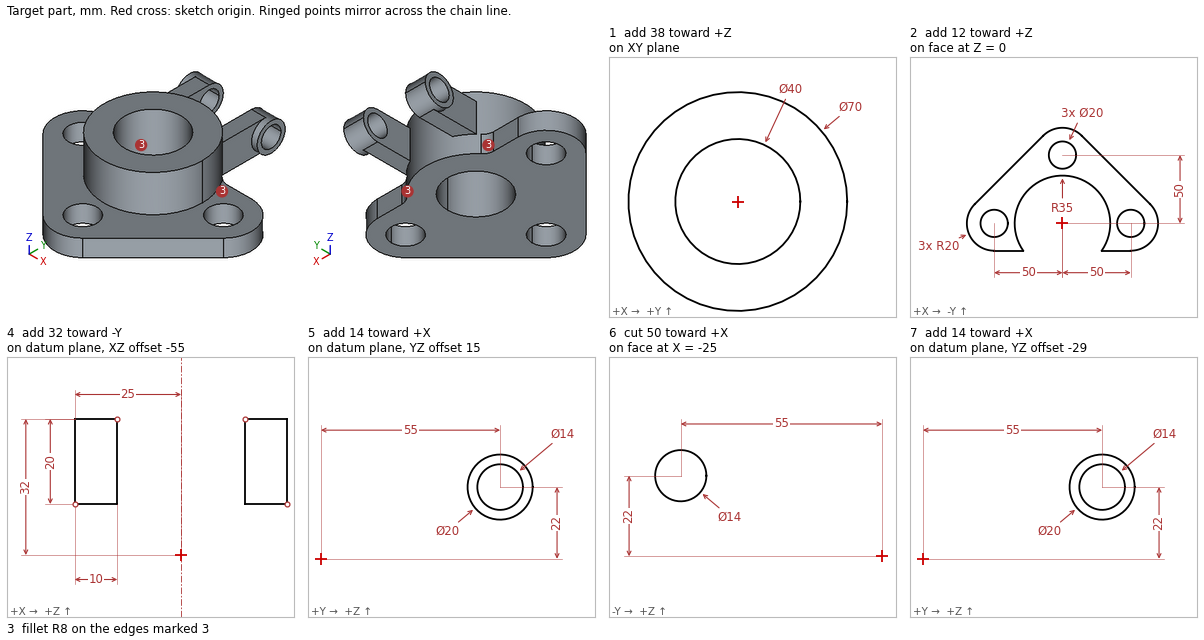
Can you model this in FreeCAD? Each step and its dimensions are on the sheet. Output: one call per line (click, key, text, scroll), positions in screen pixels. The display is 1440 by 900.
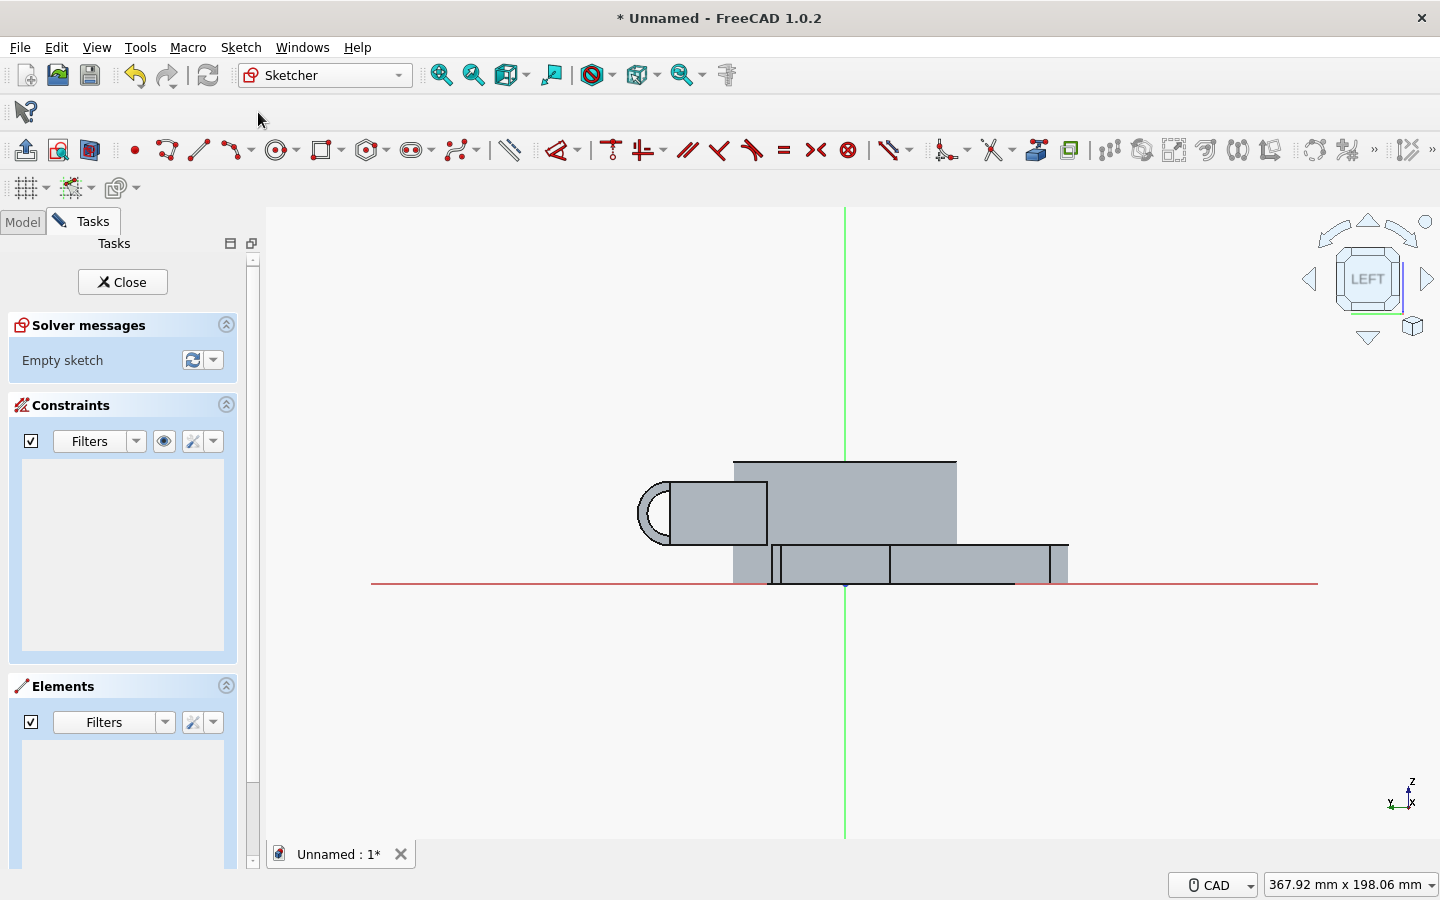
scroll(655, 512, up, 11)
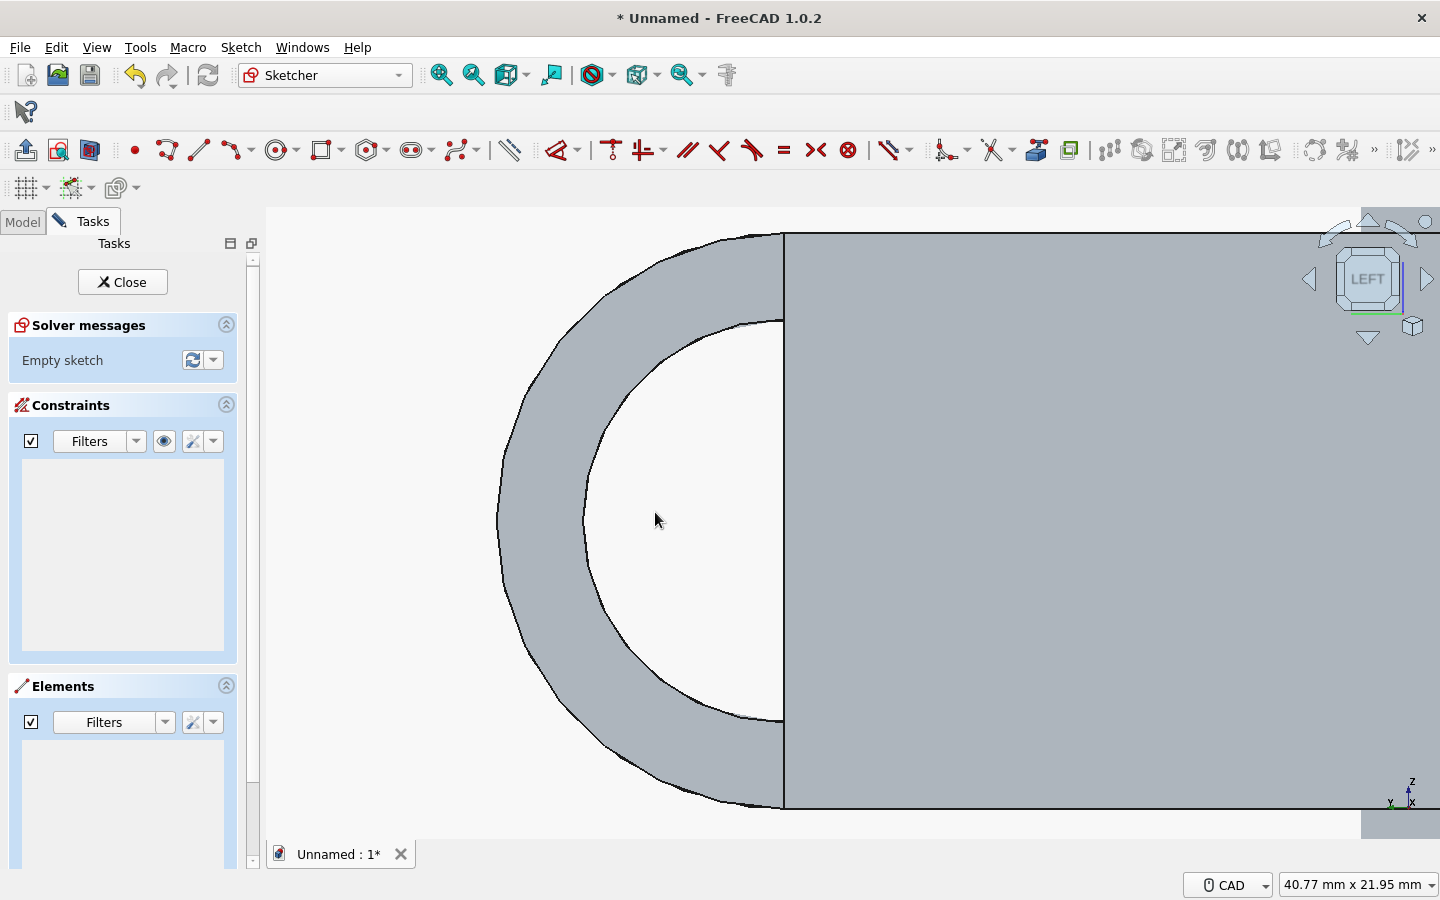
key(g)
key(c)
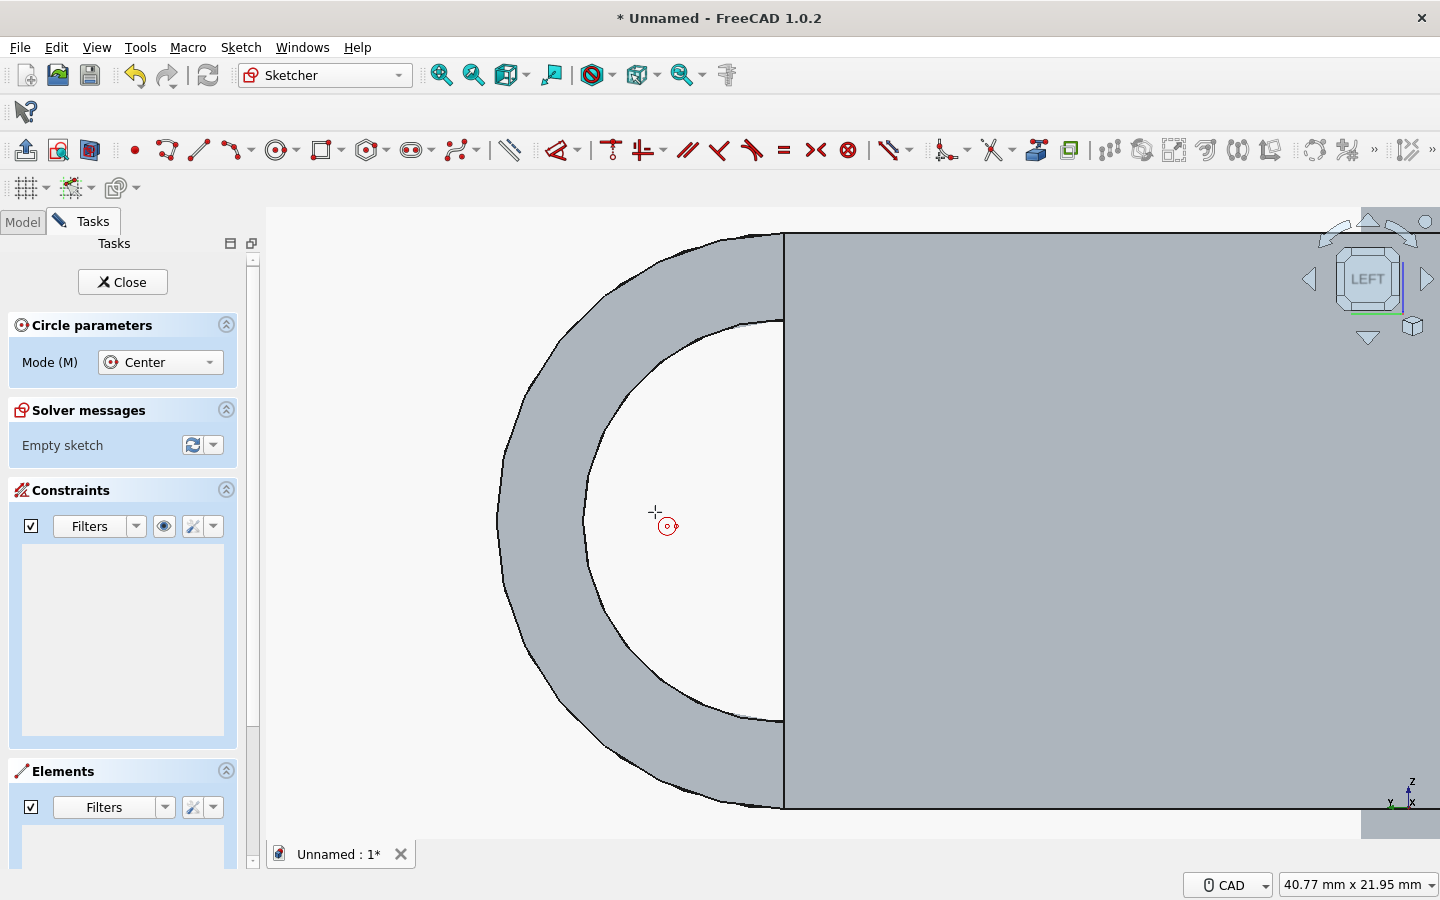
click(784, 521)
click(927, 378)
key(Escape)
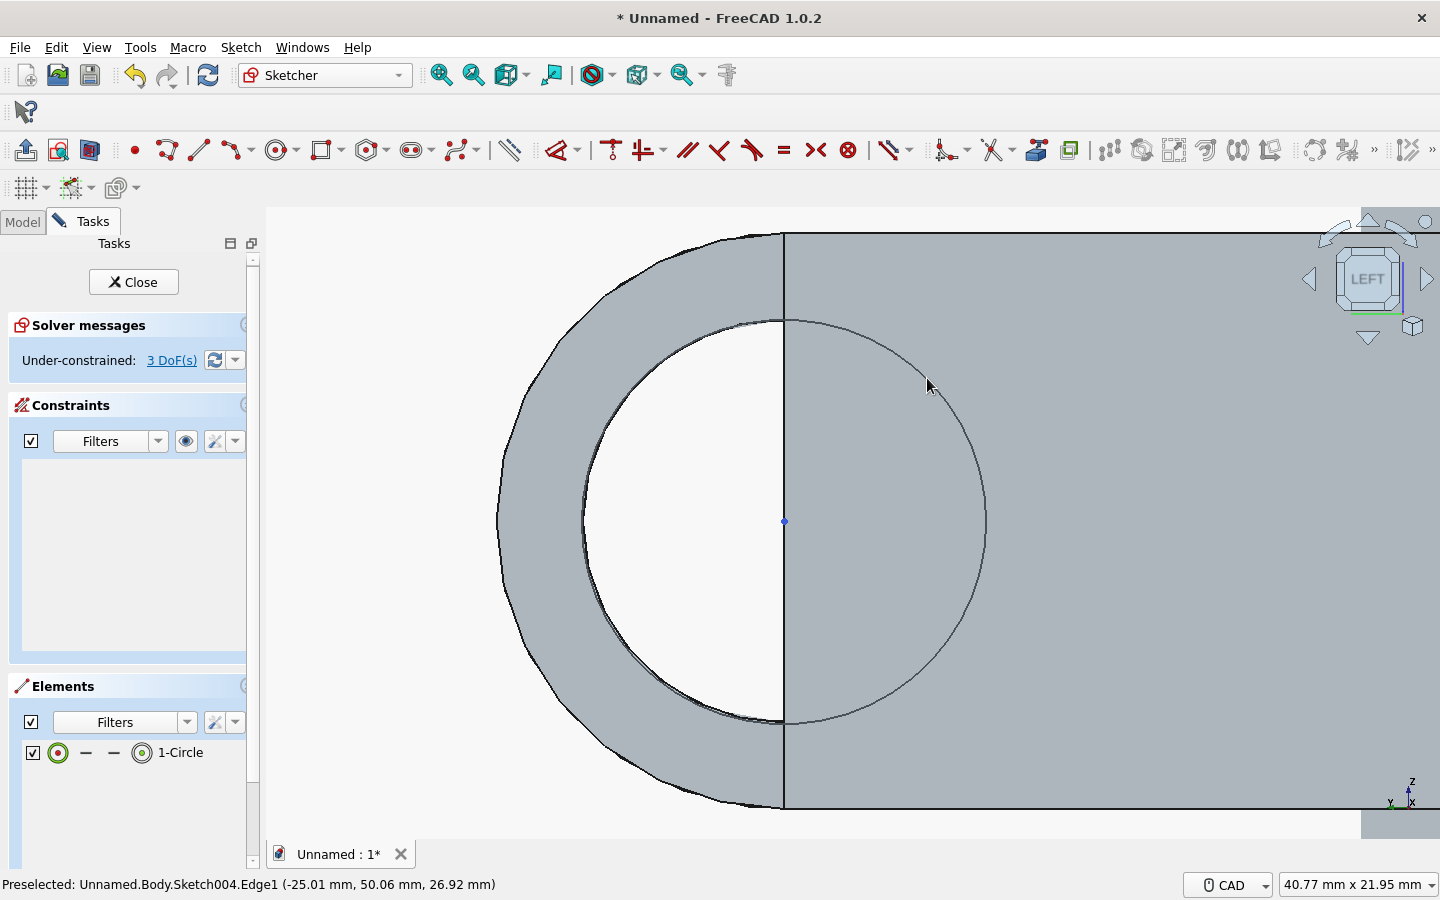
key(d)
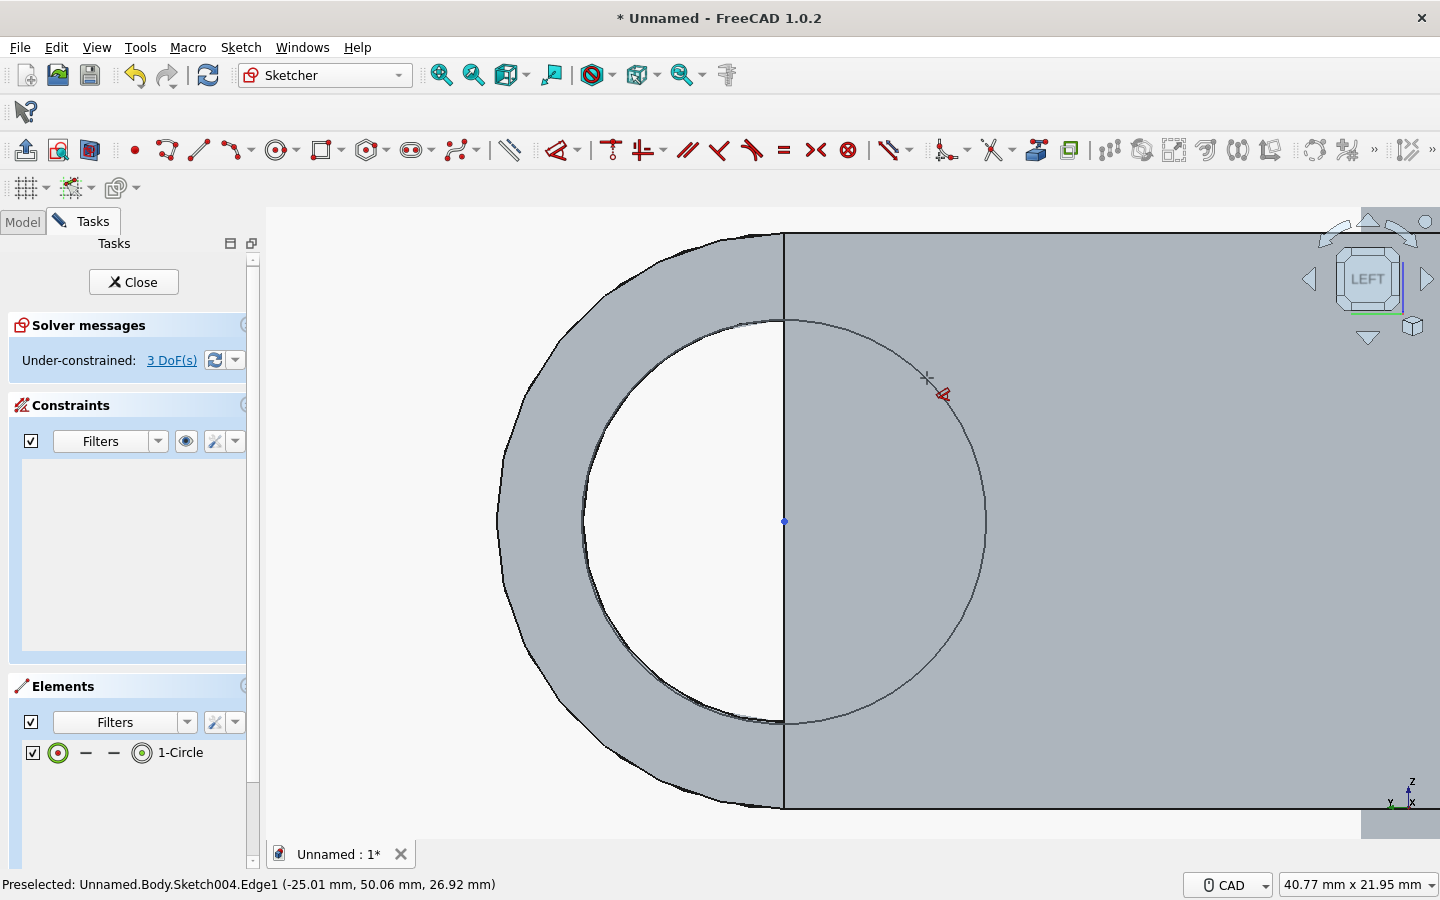
click(927, 379)
click(950, 356)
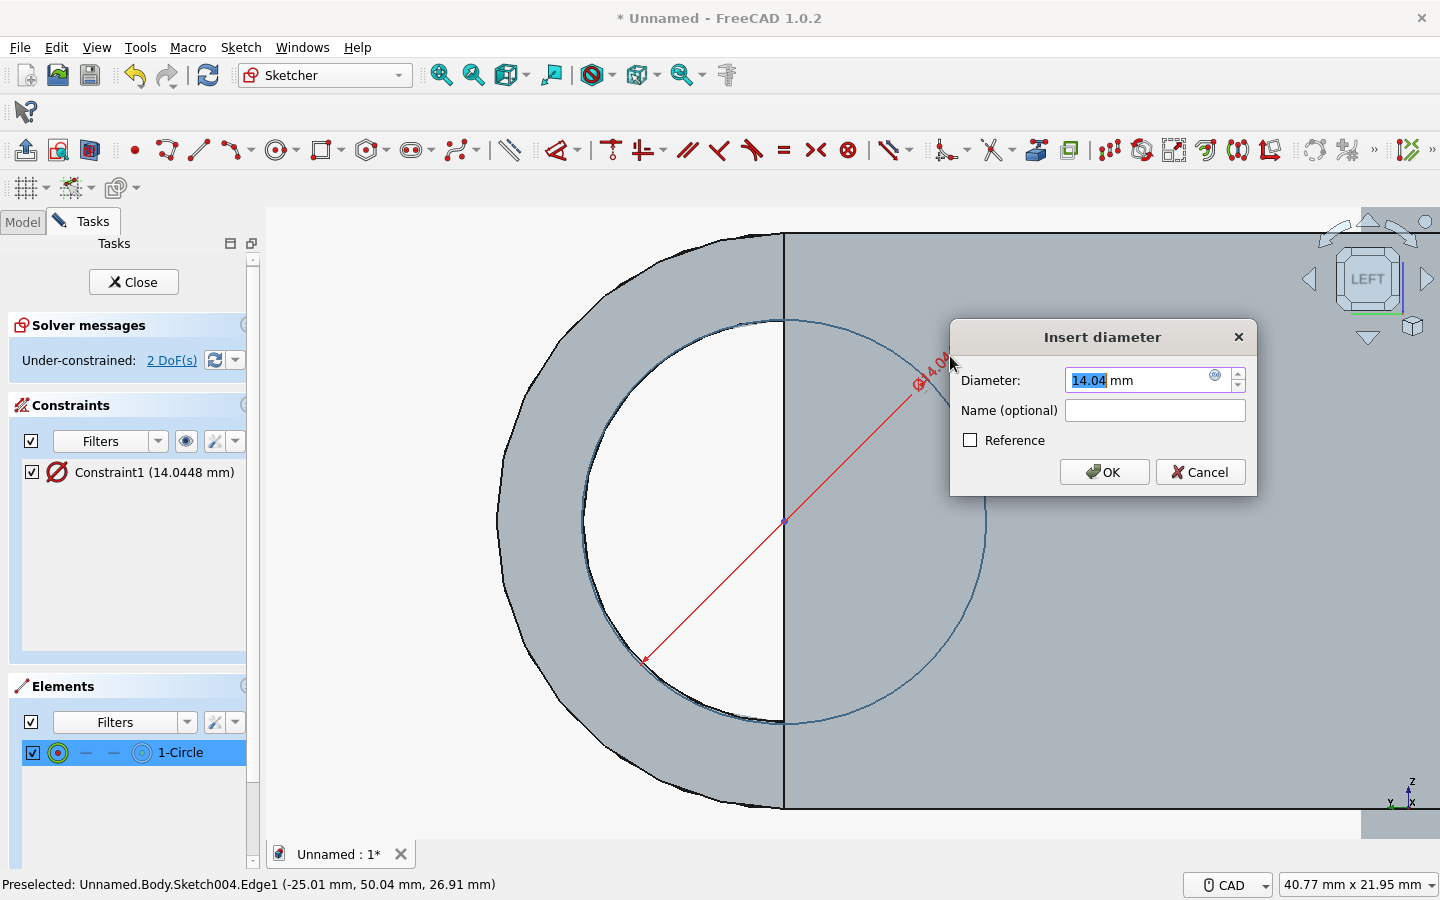
text(14)
key(Return)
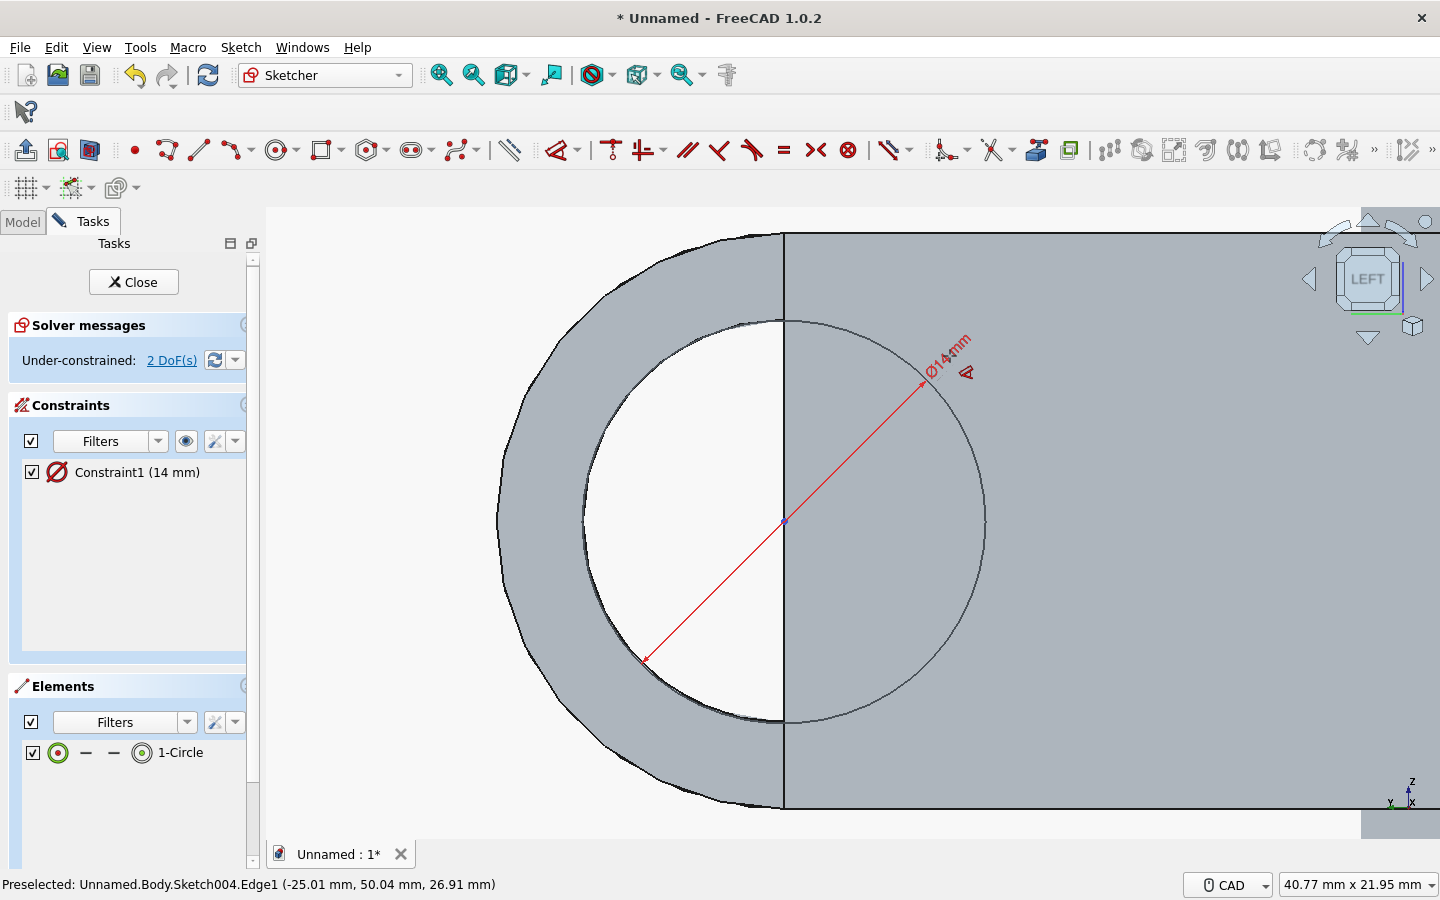
click(784, 522)
click(1029, 488)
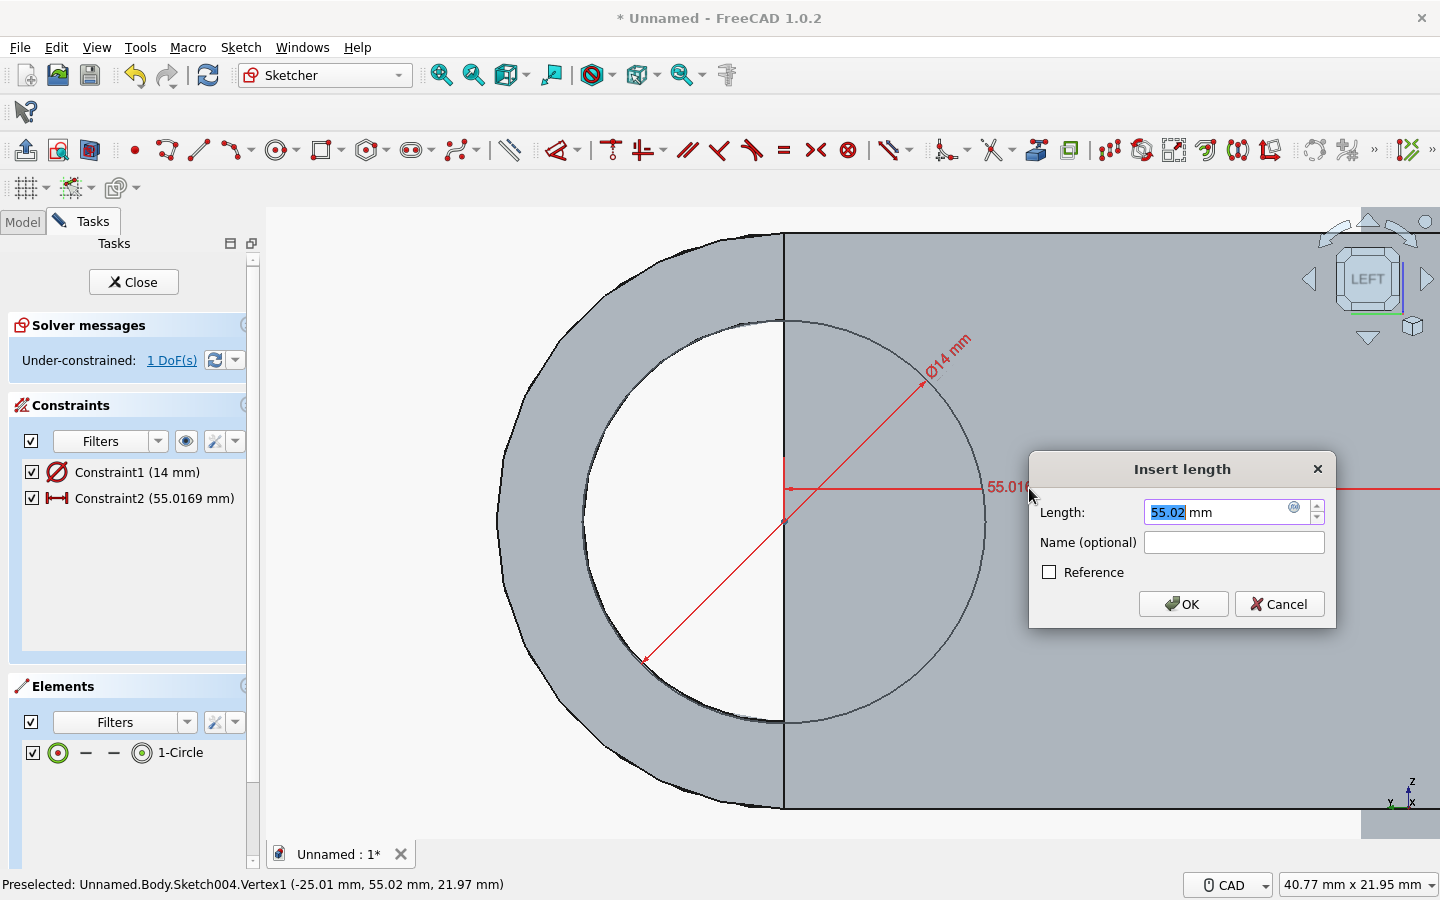
text(55)
key(Return)